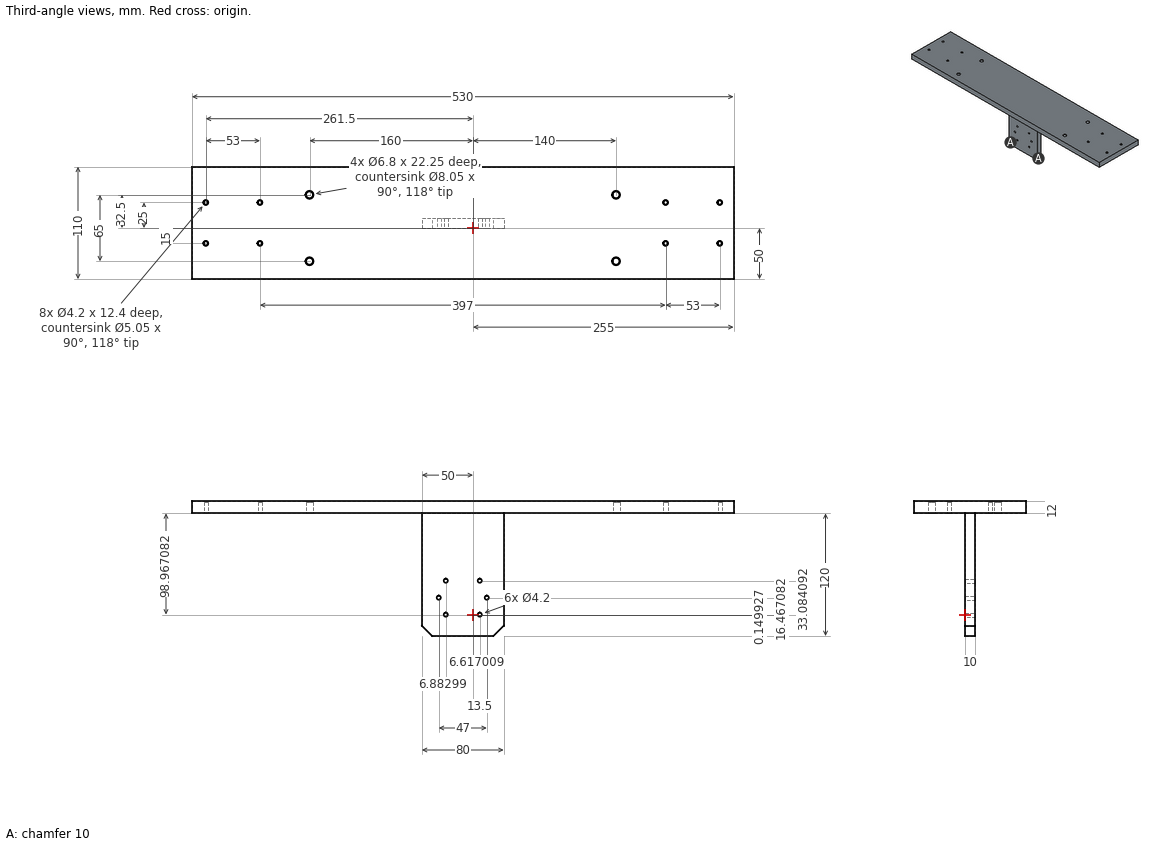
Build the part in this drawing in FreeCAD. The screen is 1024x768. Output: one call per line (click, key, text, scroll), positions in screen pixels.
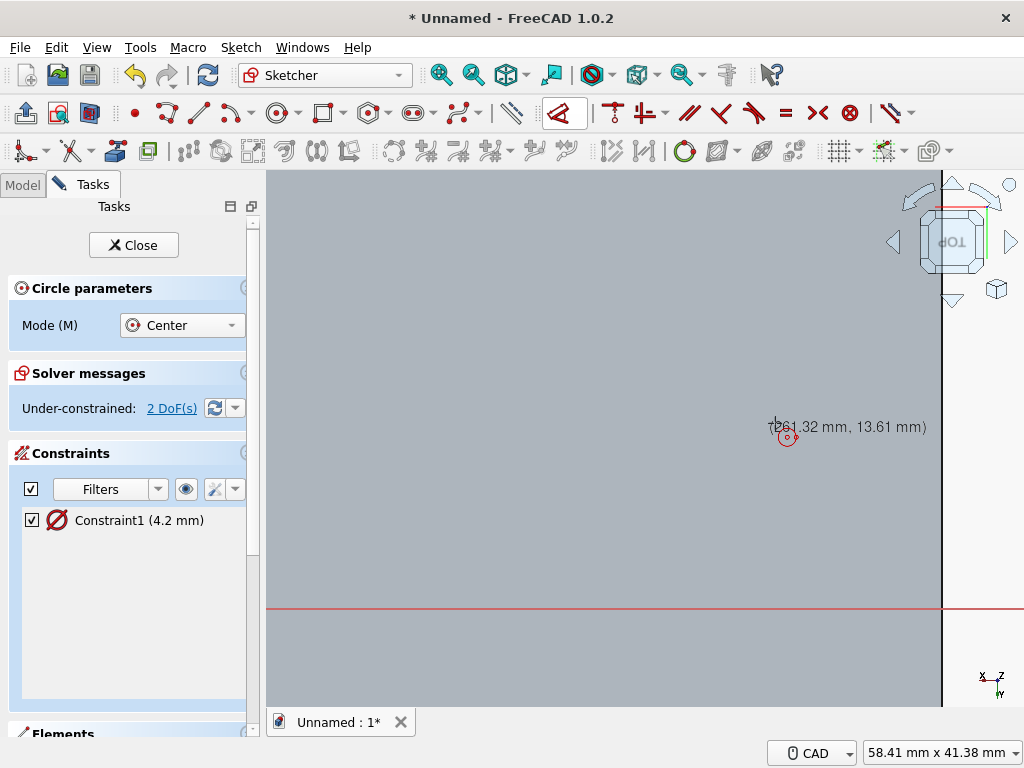
scroll(775, 423, down, 14)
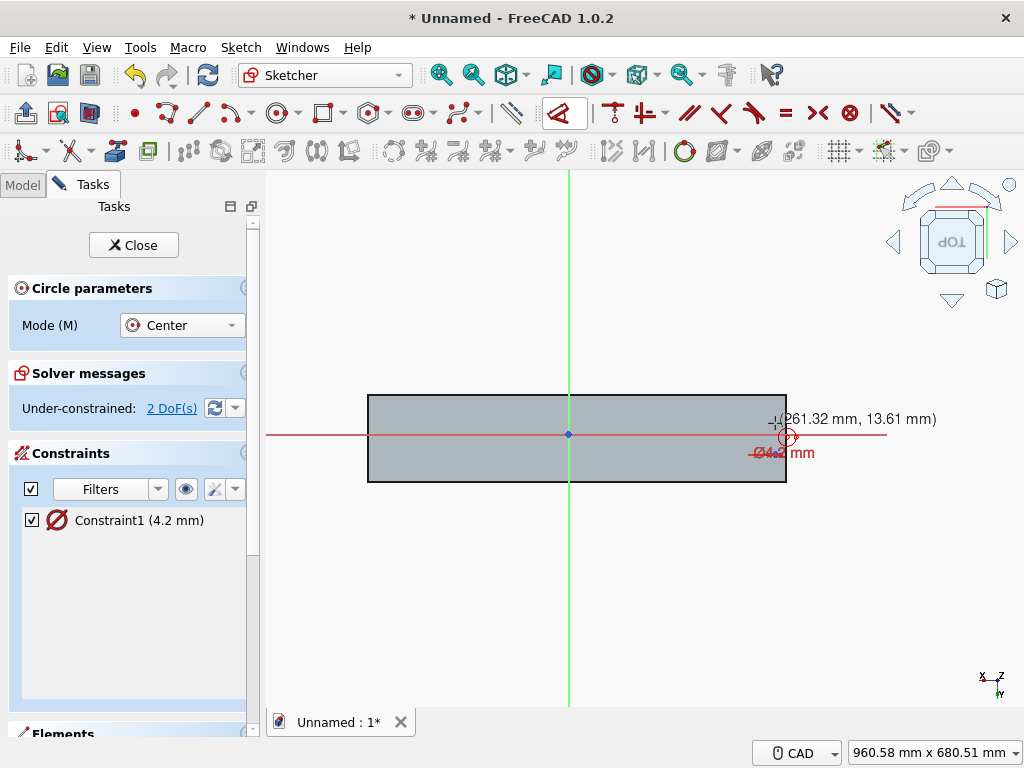
scroll(775, 423, up, 2)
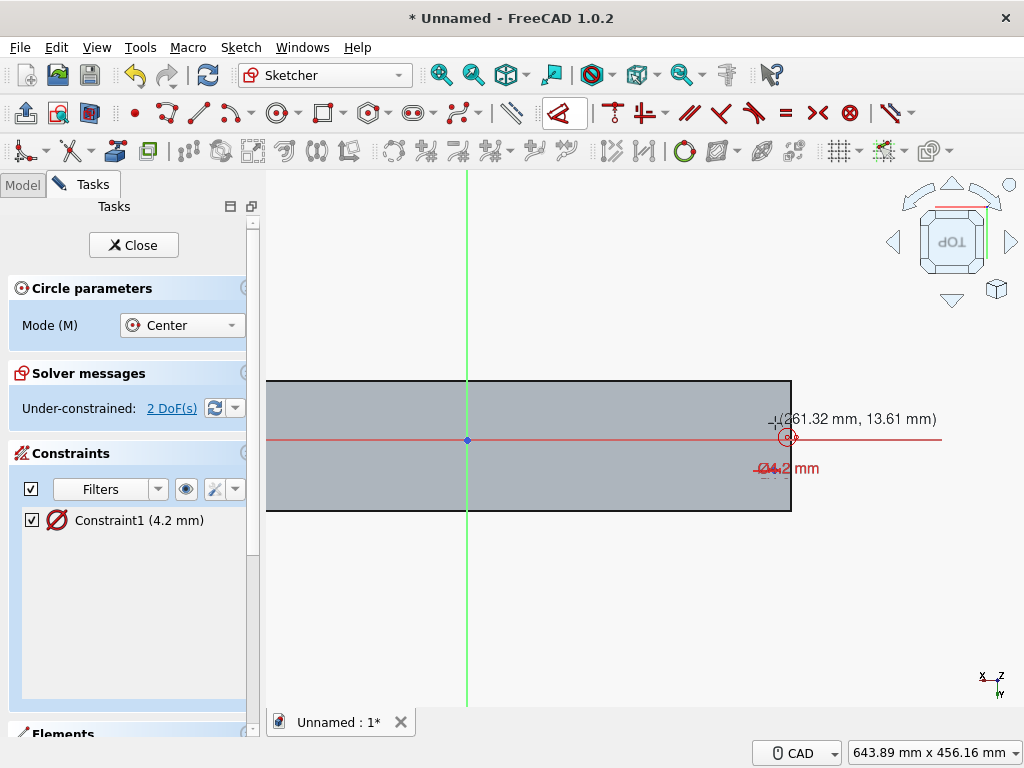
click(775, 423)
move(777, 421)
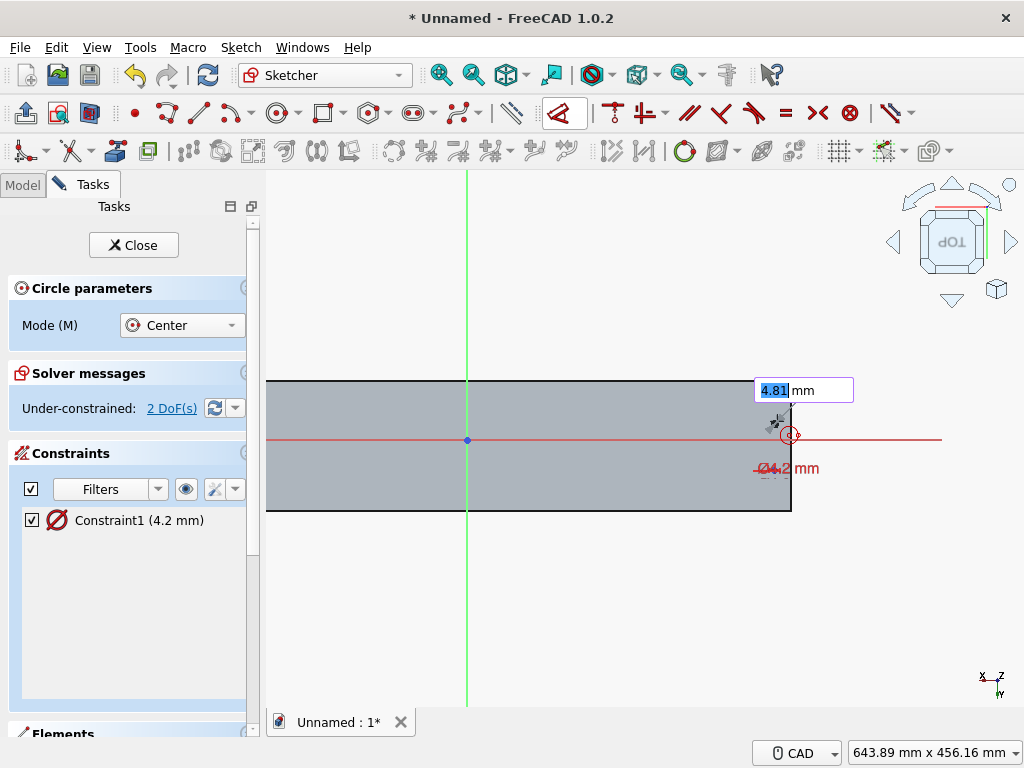
text(4.2)
key(Return)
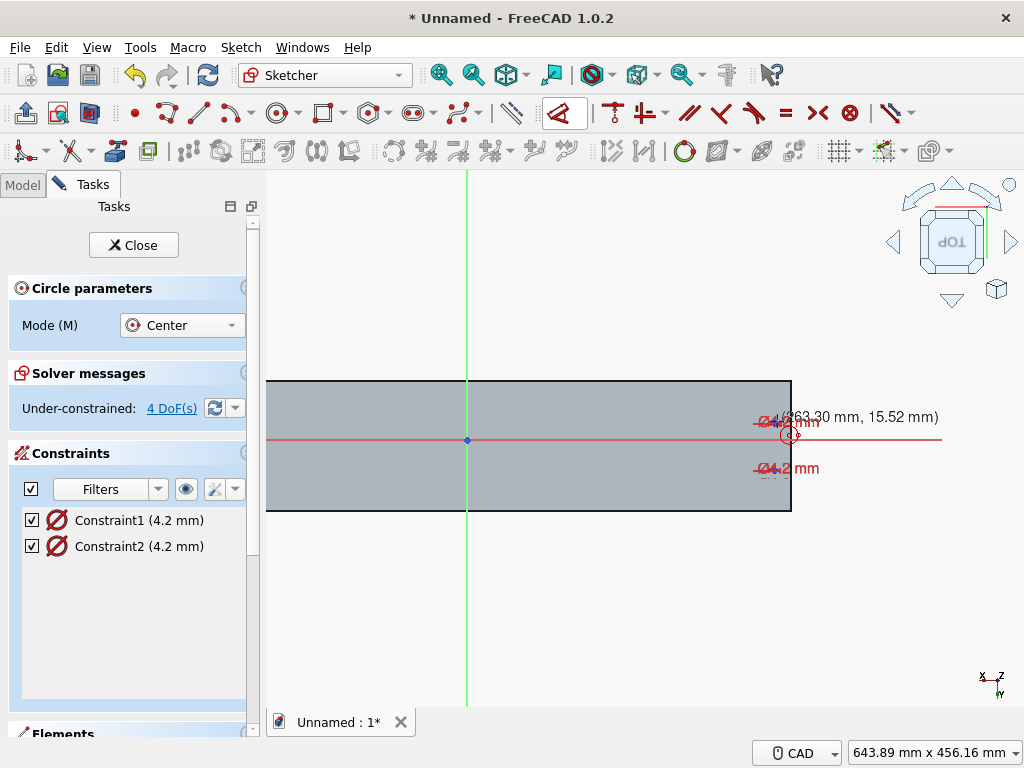
scroll(712, 470, up, 12)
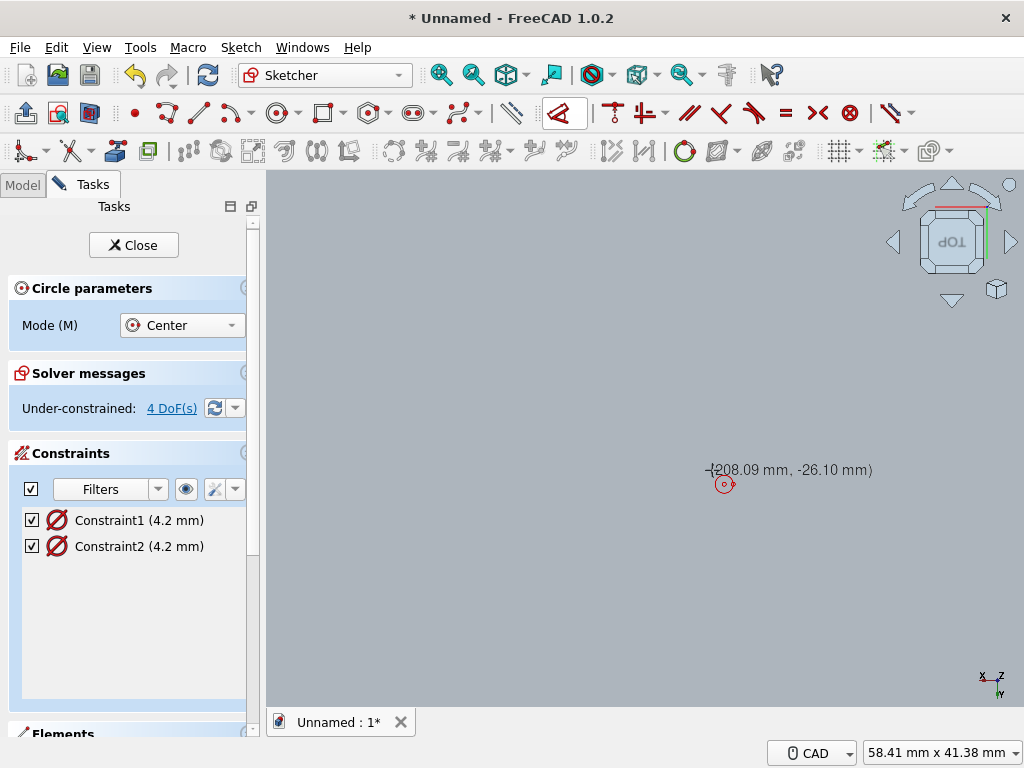
scroll(735, 454, down, 14)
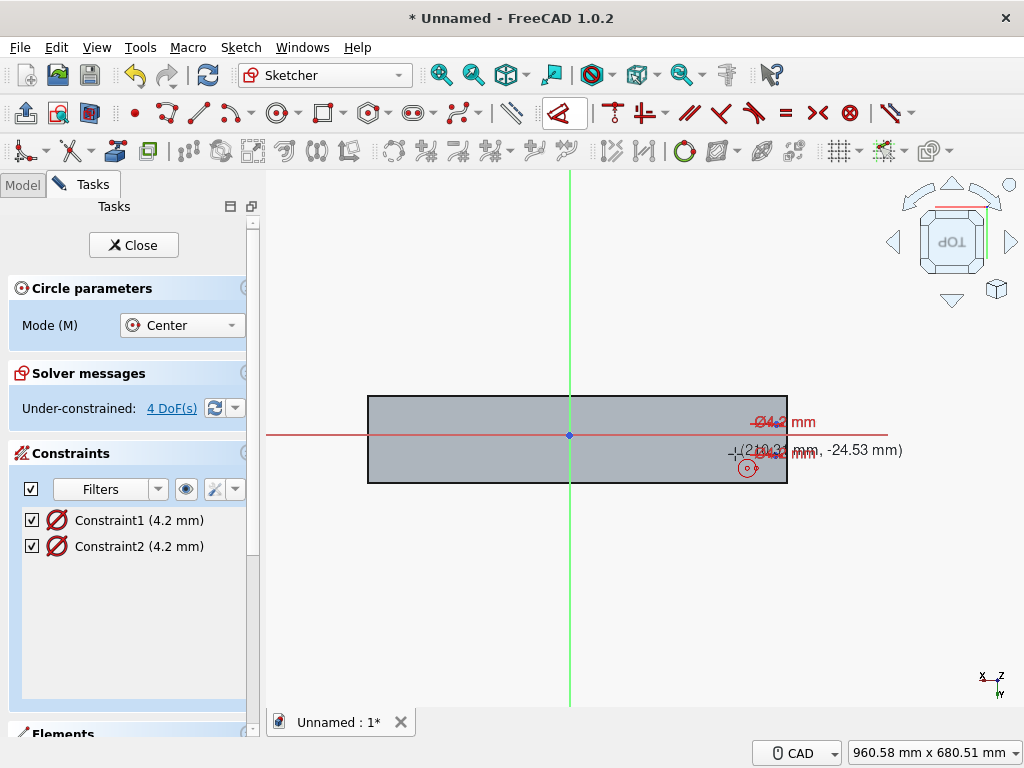
click(734, 455)
move(735, 454)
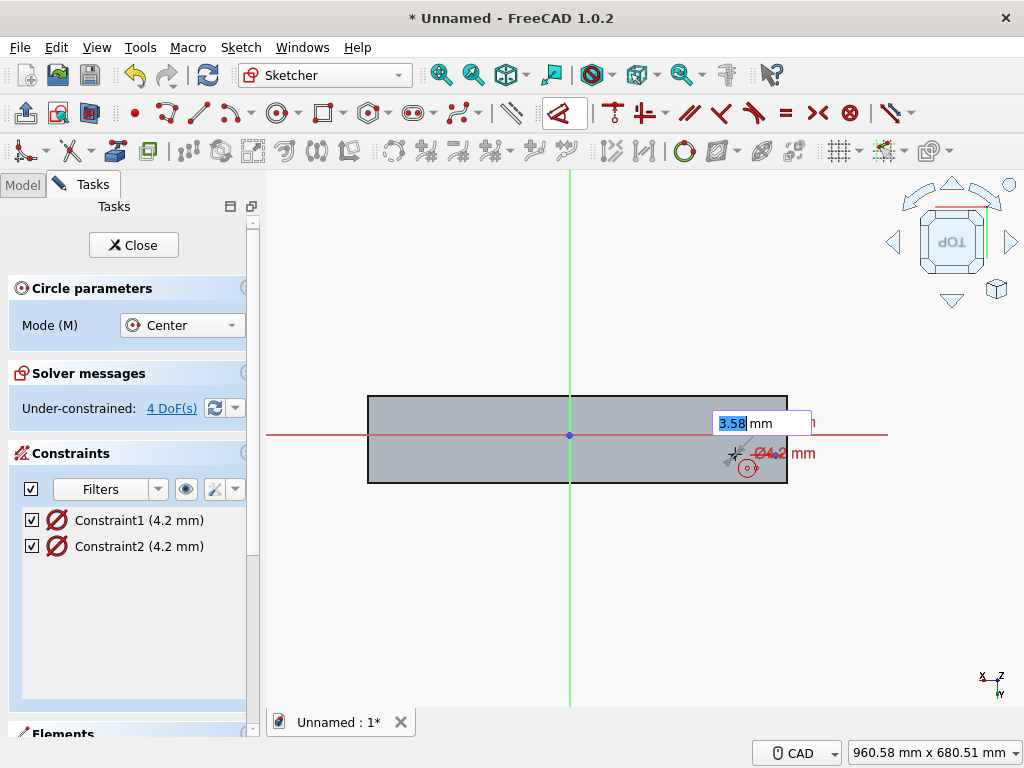
text(4.2)
key(Return)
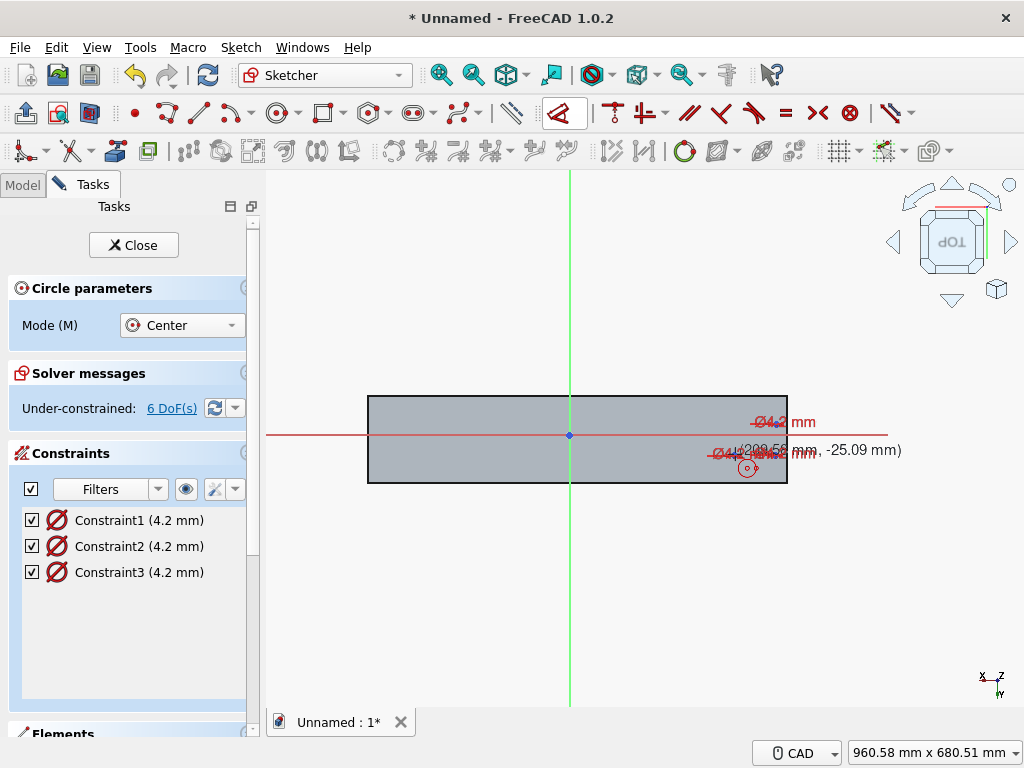
scroll(734, 423, up, 14)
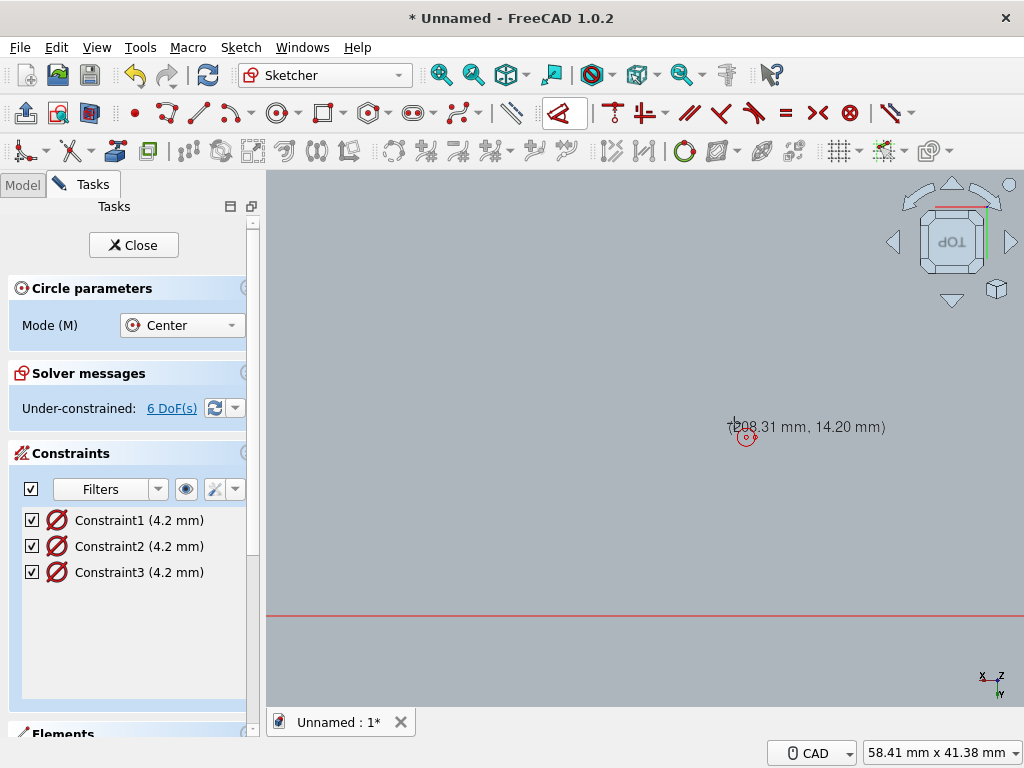
scroll(734, 423, down, 14)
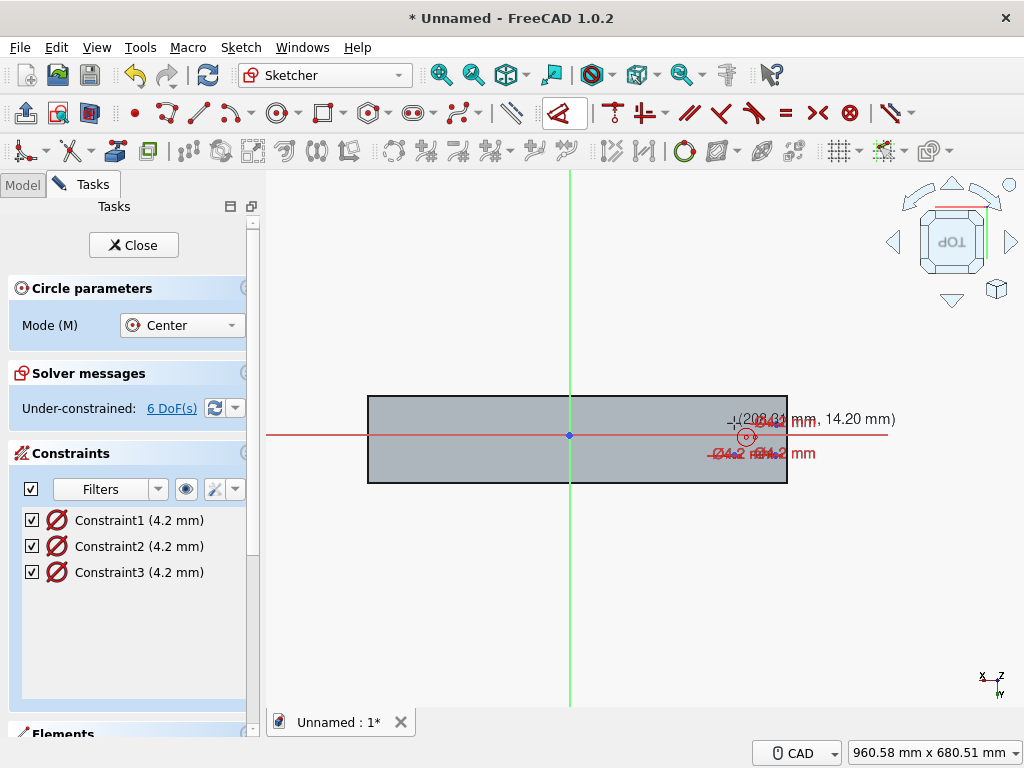
scroll(734, 423, up, 2)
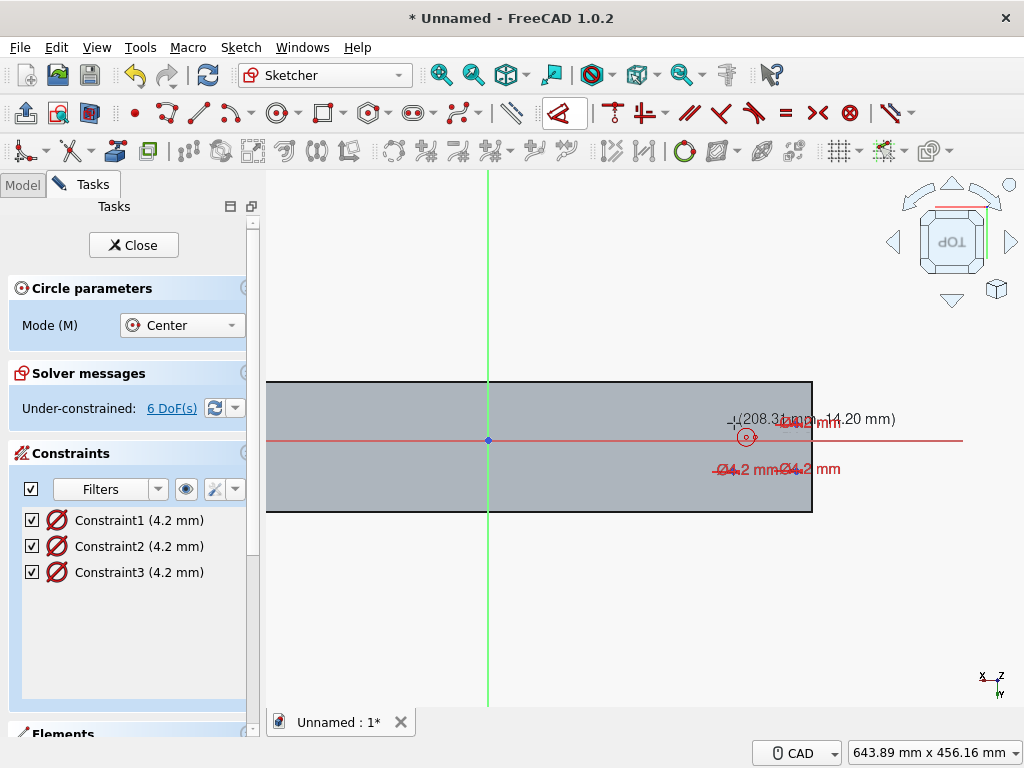
click(734, 423)
move(736, 422)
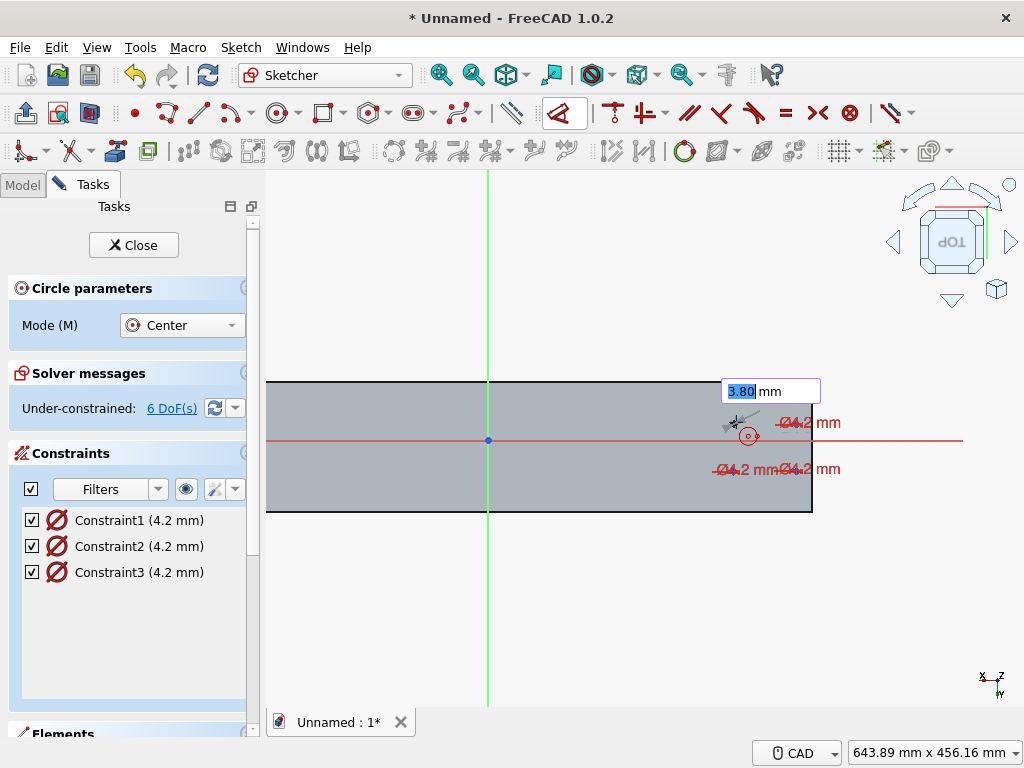
text(4.2)
key(Return)